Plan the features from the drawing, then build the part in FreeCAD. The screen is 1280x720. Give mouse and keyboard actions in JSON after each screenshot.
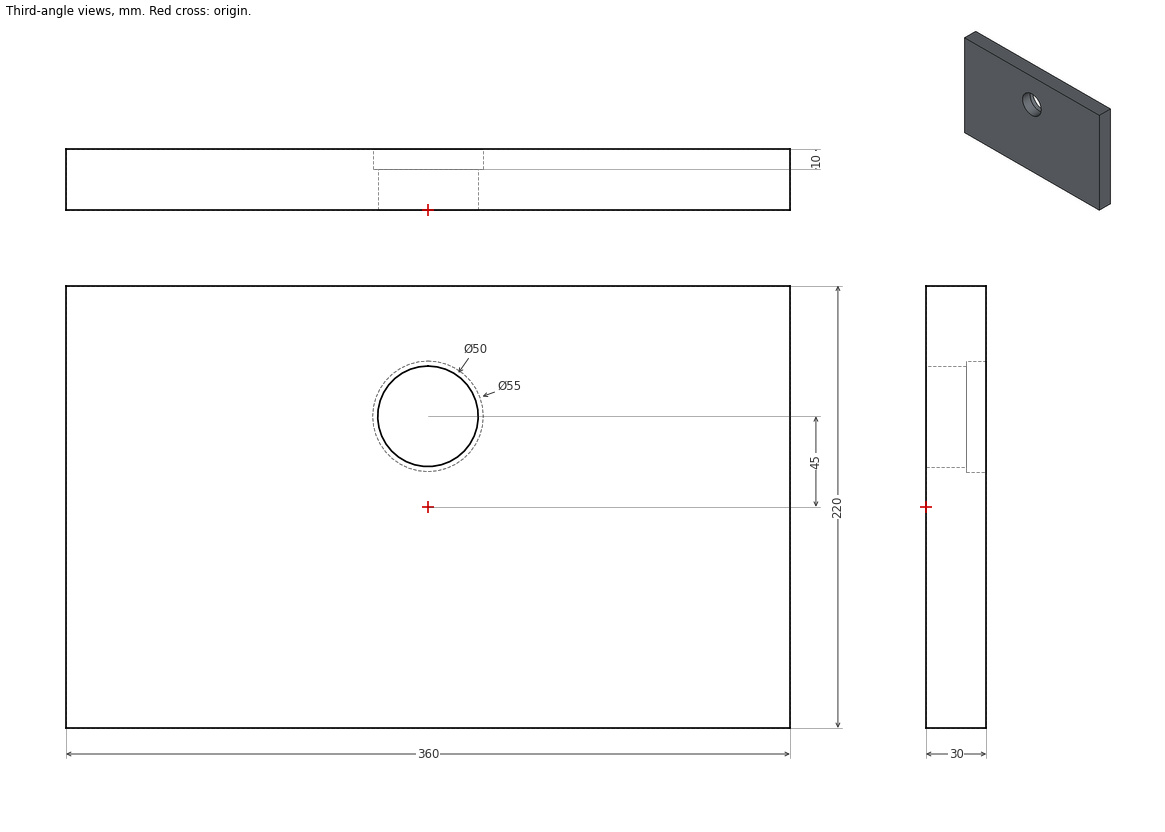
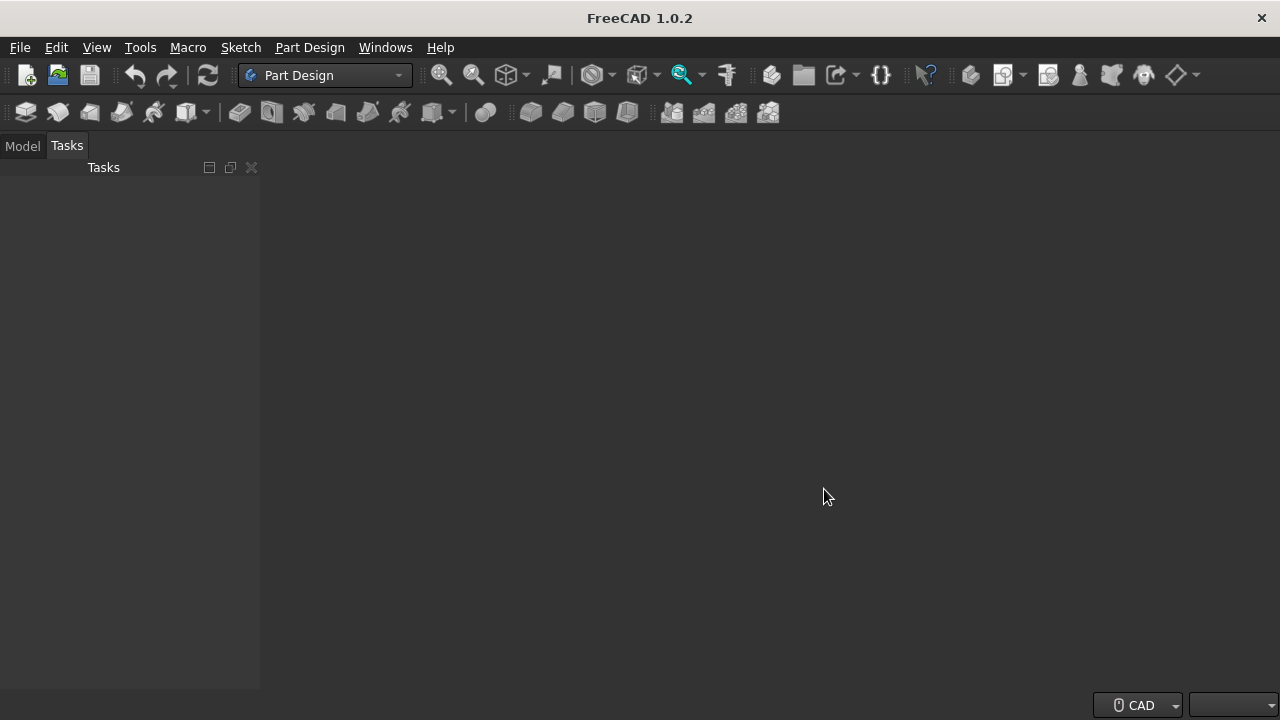
{"action": "left_click", "coordinate": [26, 76]}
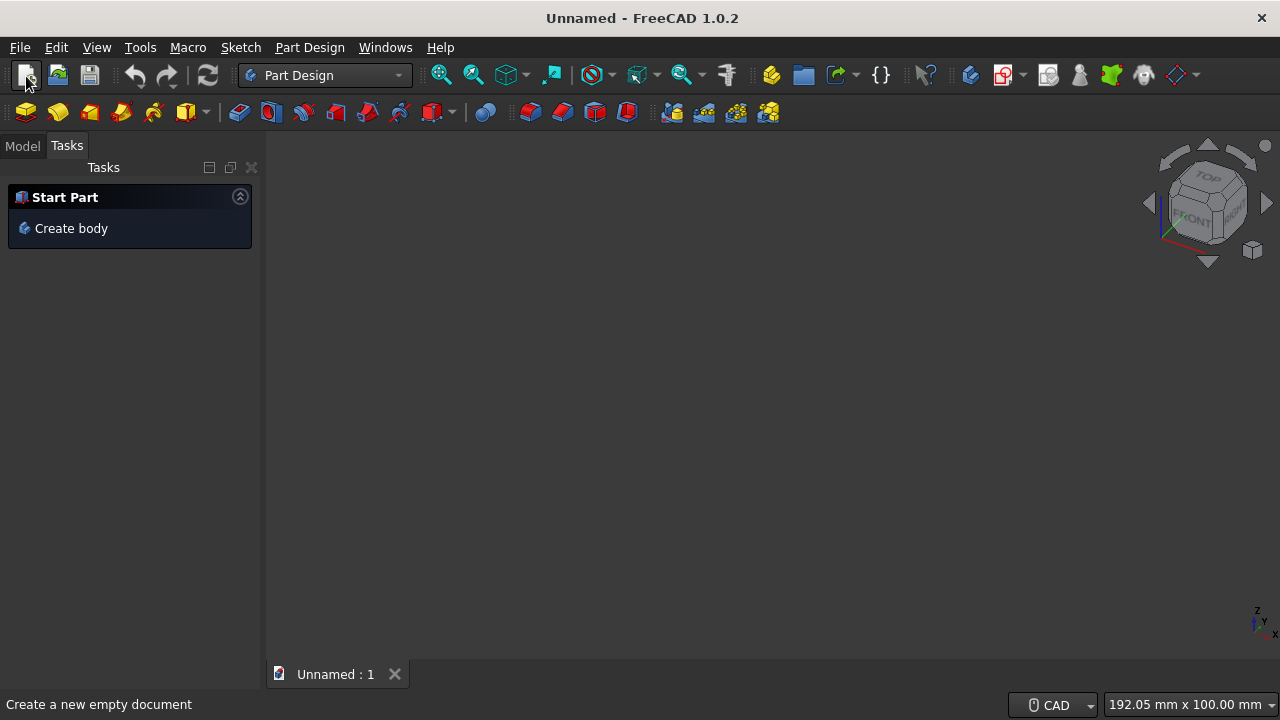
{"action": "left_click", "coordinate": [1004, 76]}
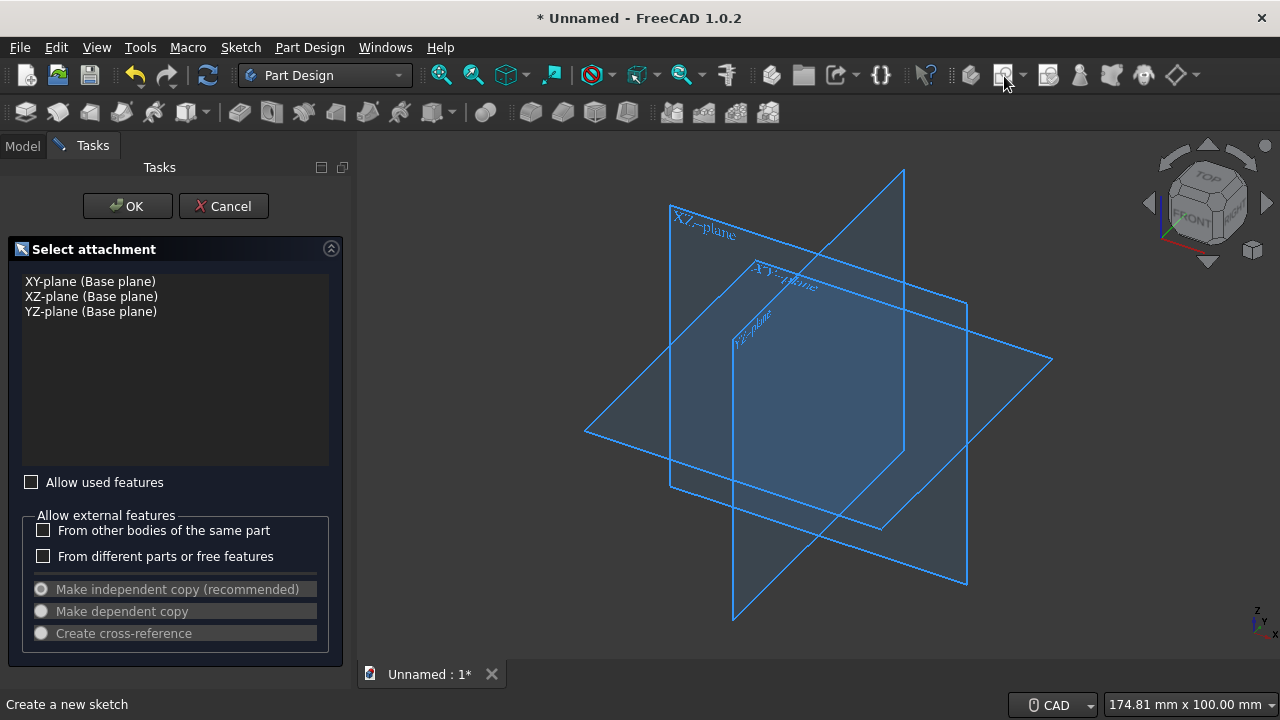
{"action": "left_click", "coordinate": [82, 296]}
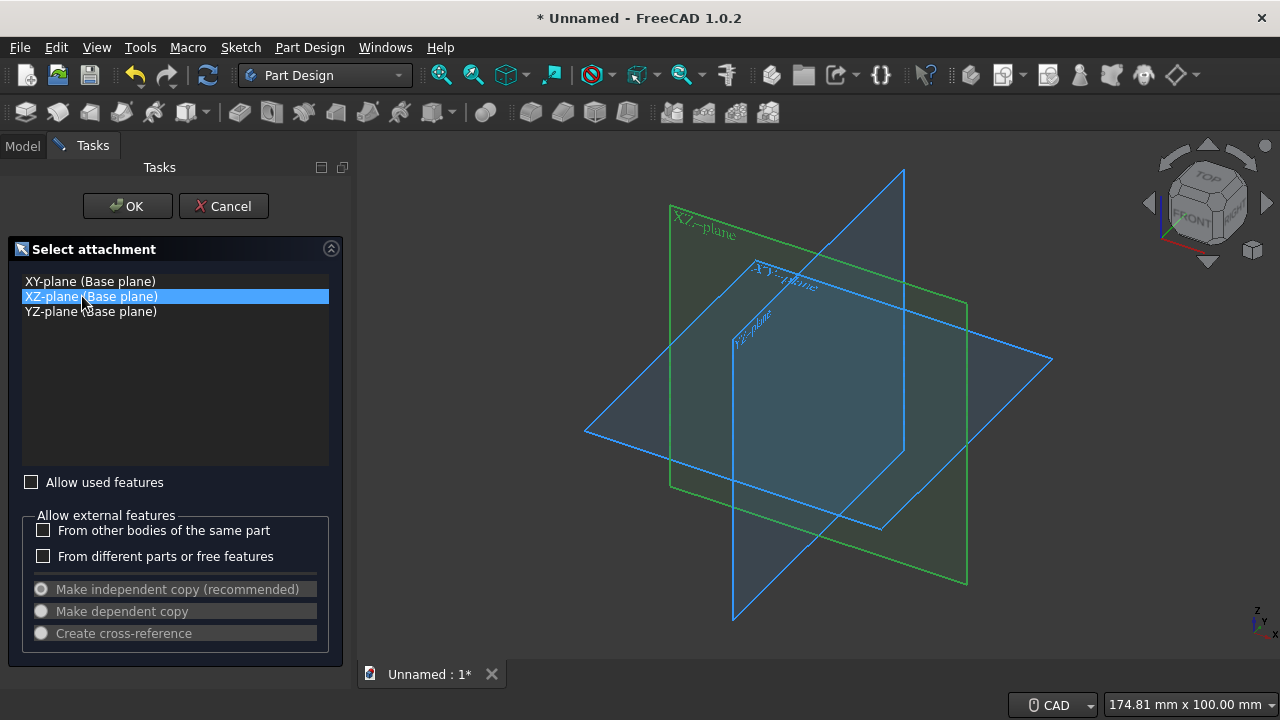
{"action": "left_click", "coordinate": [128, 206]}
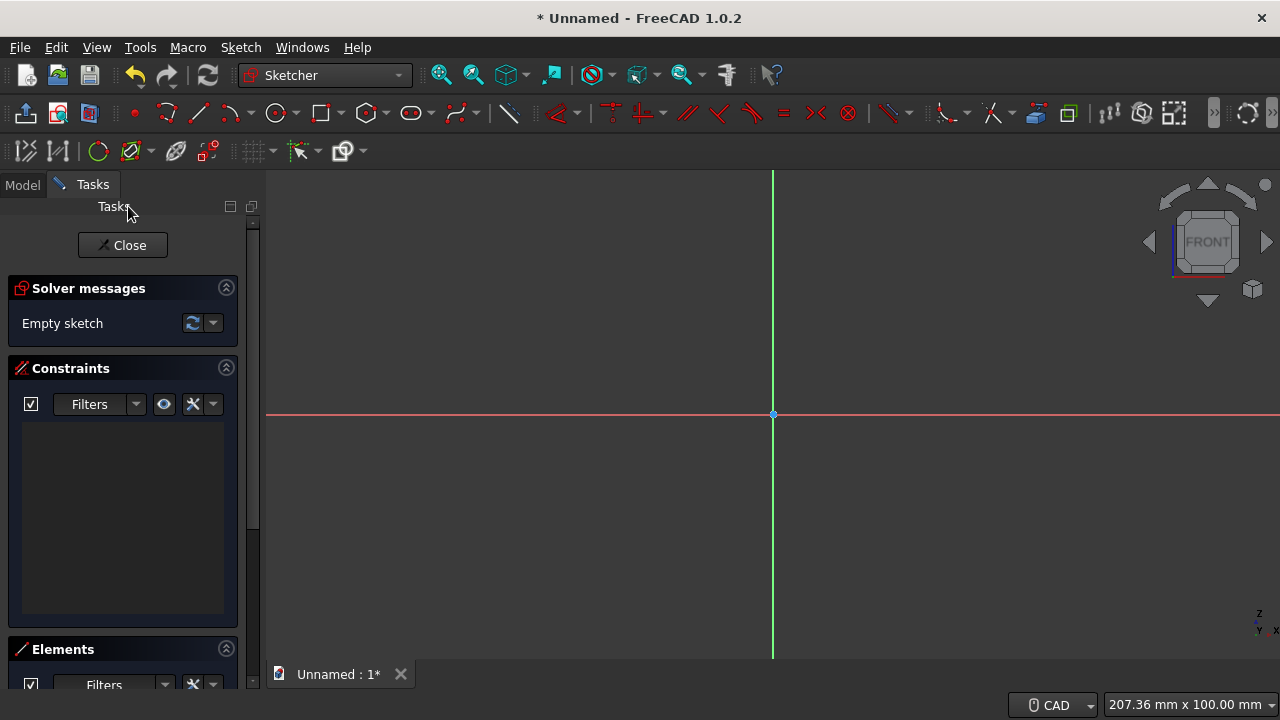
{"action": "scroll", "coordinate": [675, 414], "scroll_direction": "down", "scroll_amount": 6}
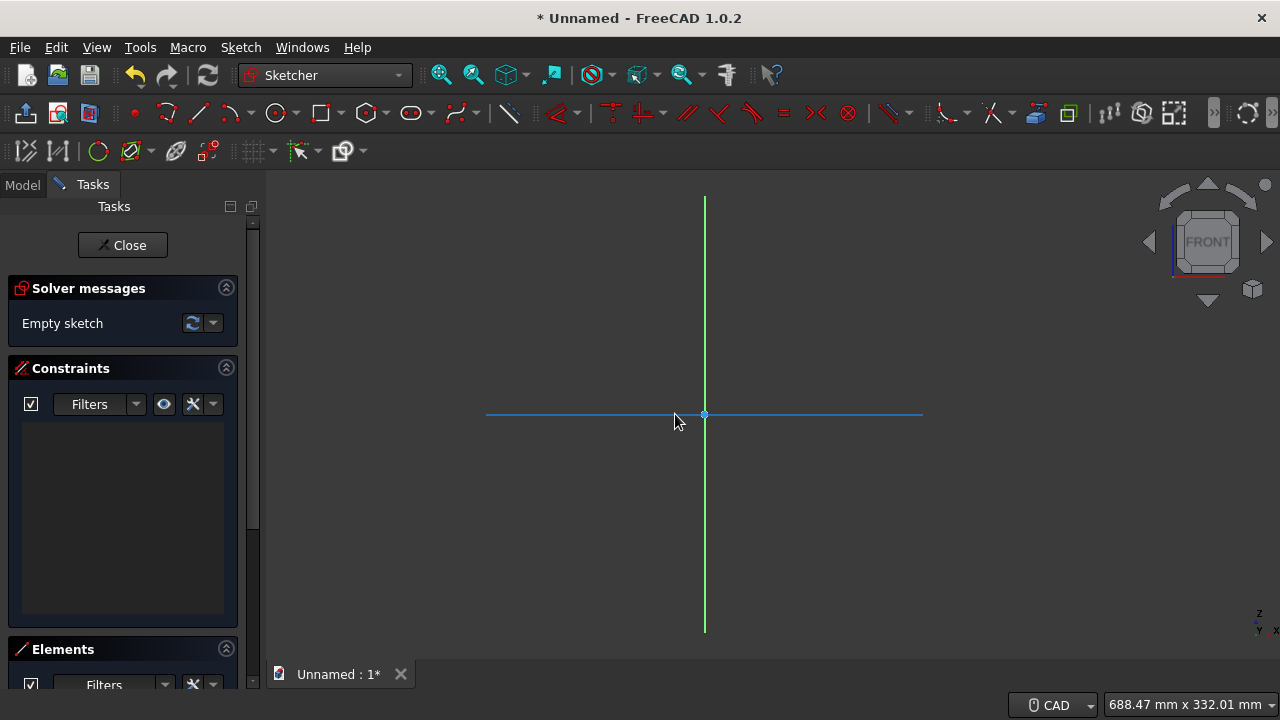
{"action": "key", "text": "g v"}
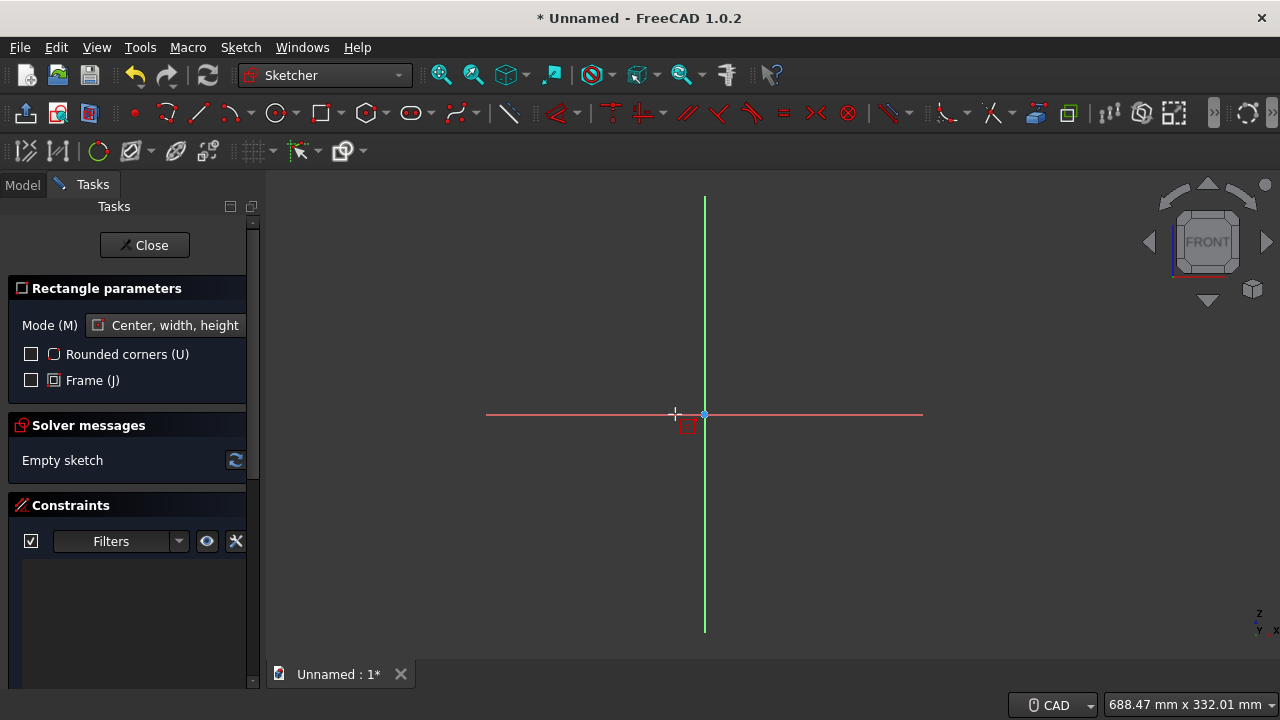
{"action": "left_click", "coordinate": [705, 414]}
{"action": "mouse_move", "coordinate": [970, 252]}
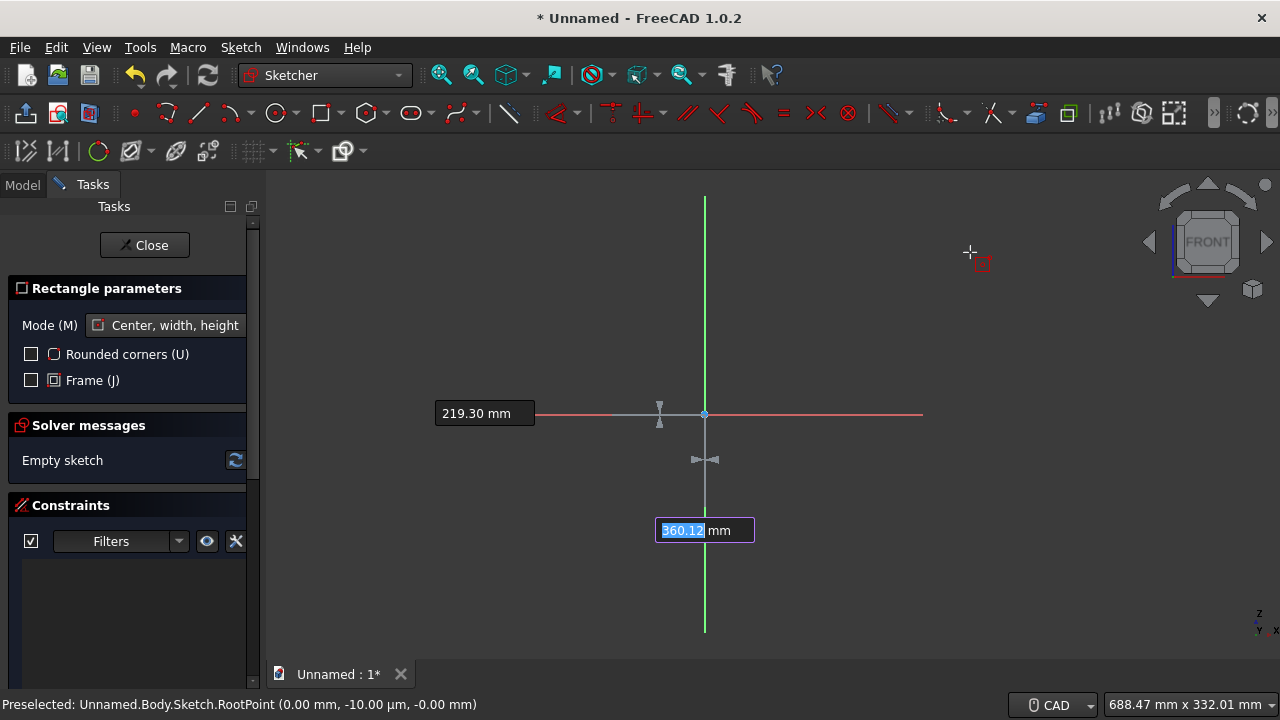
{"action": "type", "text": "360"}
{"action": "key", "text": "Tab"}
{"action": "type", "text": "220"}
{"action": "key", "text": "Return"}
{"action": "key", "text": "Escape"}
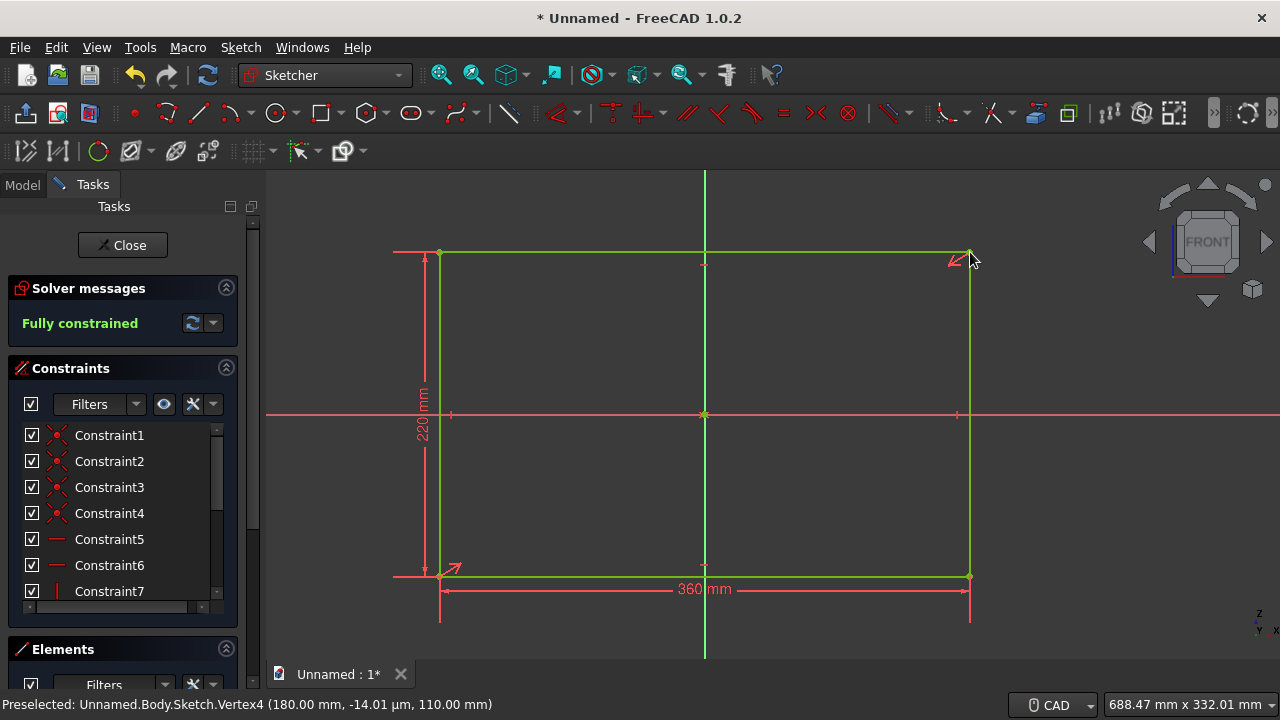
{"action": "left_click", "coordinate": [123, 245]}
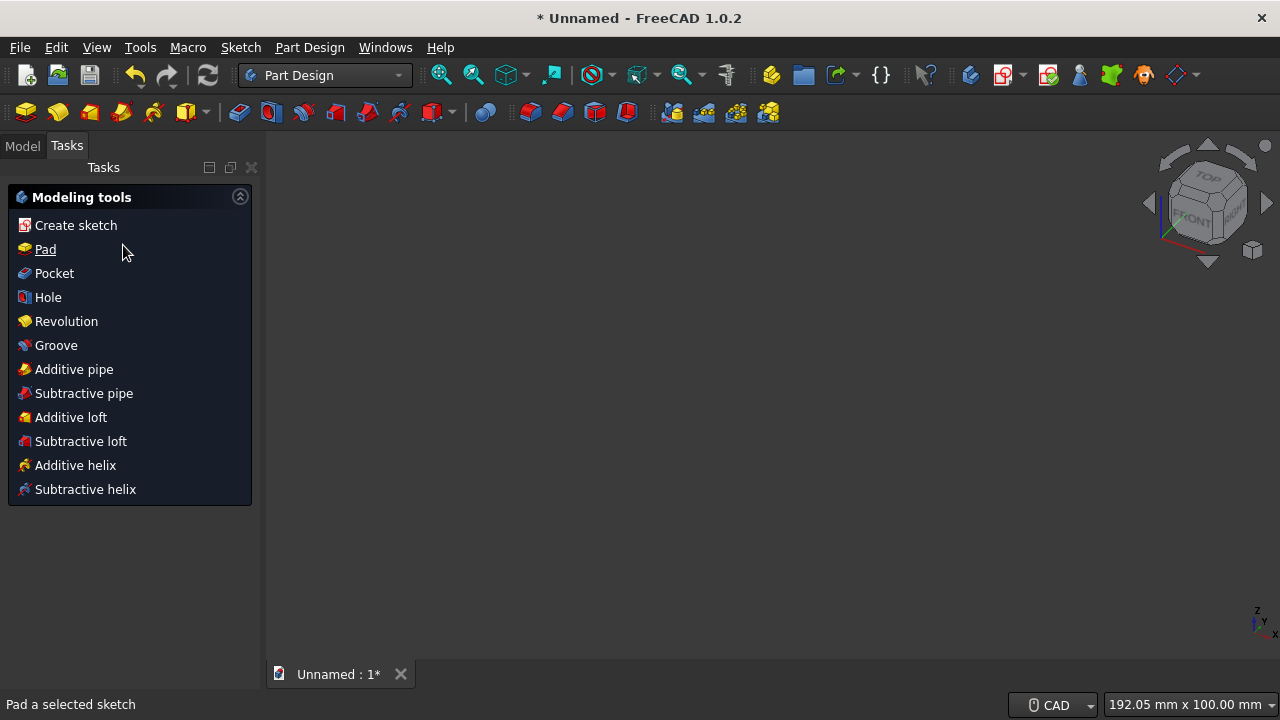
{"action": "left_click", "coordinate": [26, 112]}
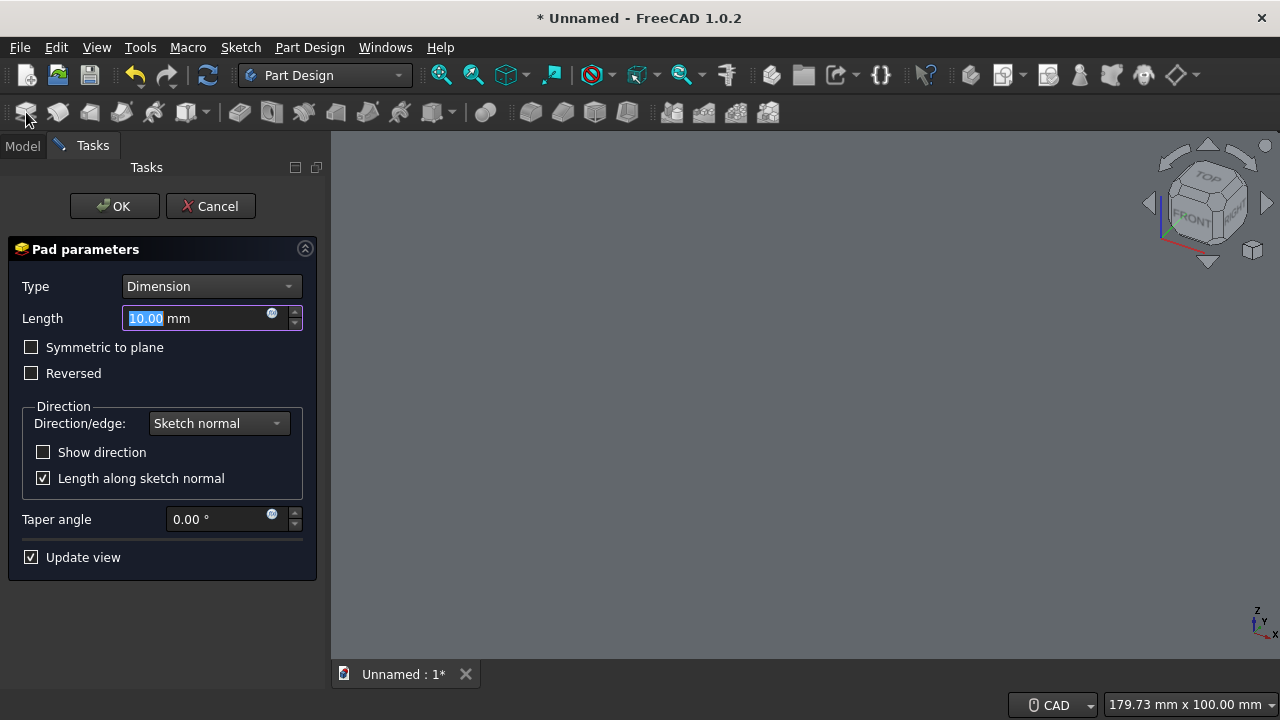
{"action": "type", "text": "30"}
{"action": "key", "text": "Tab"}